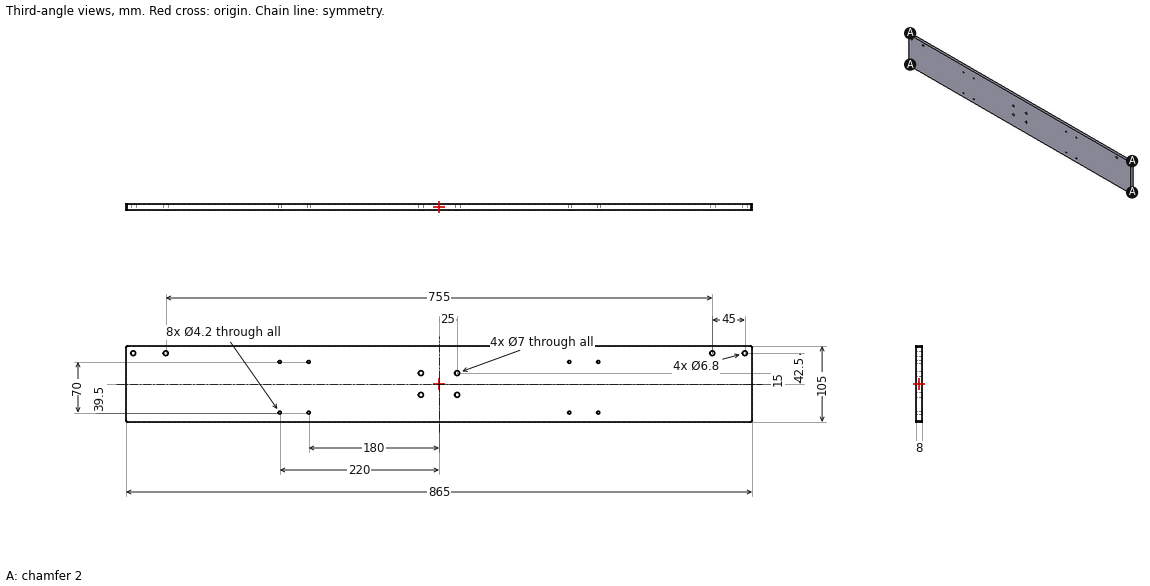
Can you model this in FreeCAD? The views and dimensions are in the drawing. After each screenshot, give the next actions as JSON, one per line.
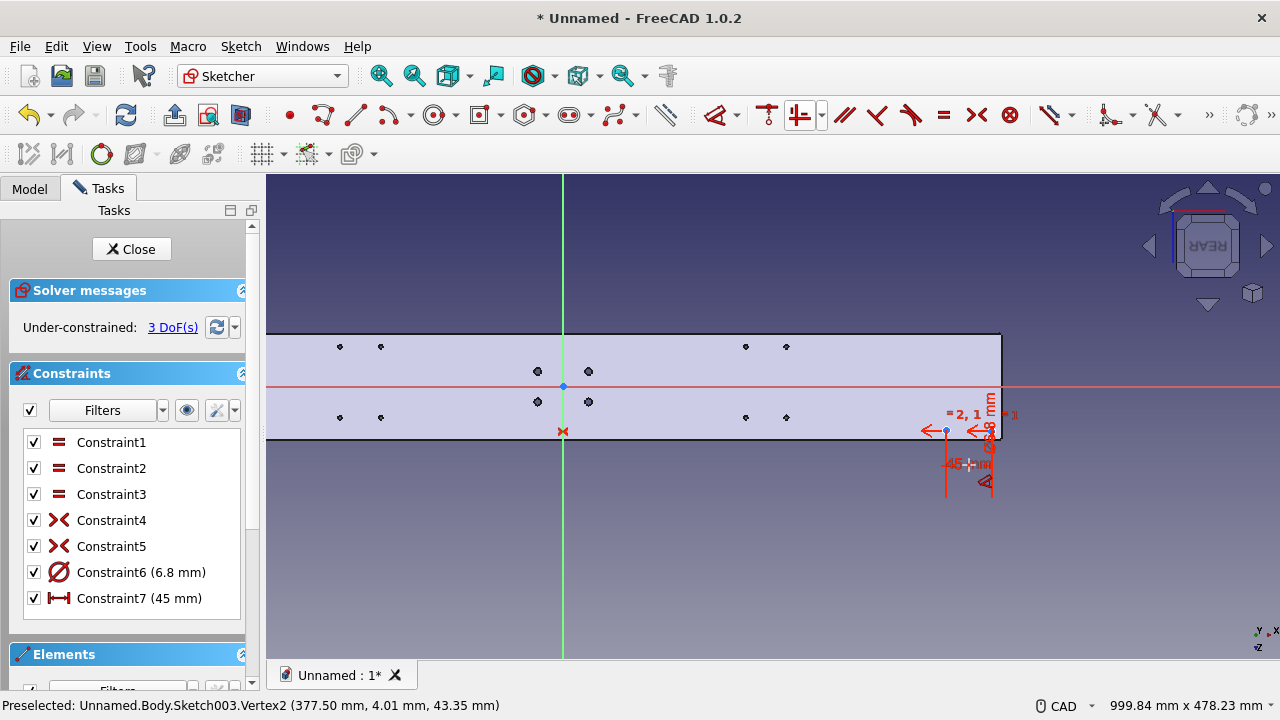
{"action": "left_click", "coordinate": [992, 431]}
{"action": "left_click", "coordinate": [529, 409]}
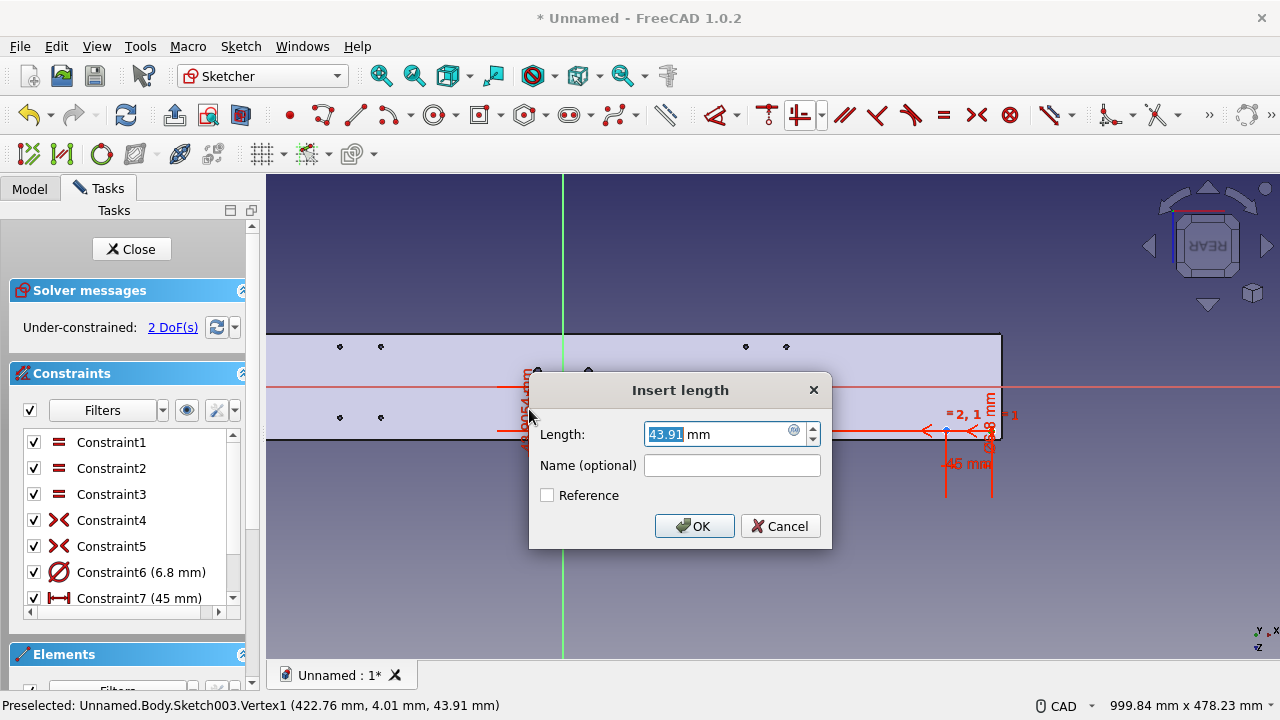
{"action": "type", "text": "42.5"}
{"action": "key", "text": "Return"}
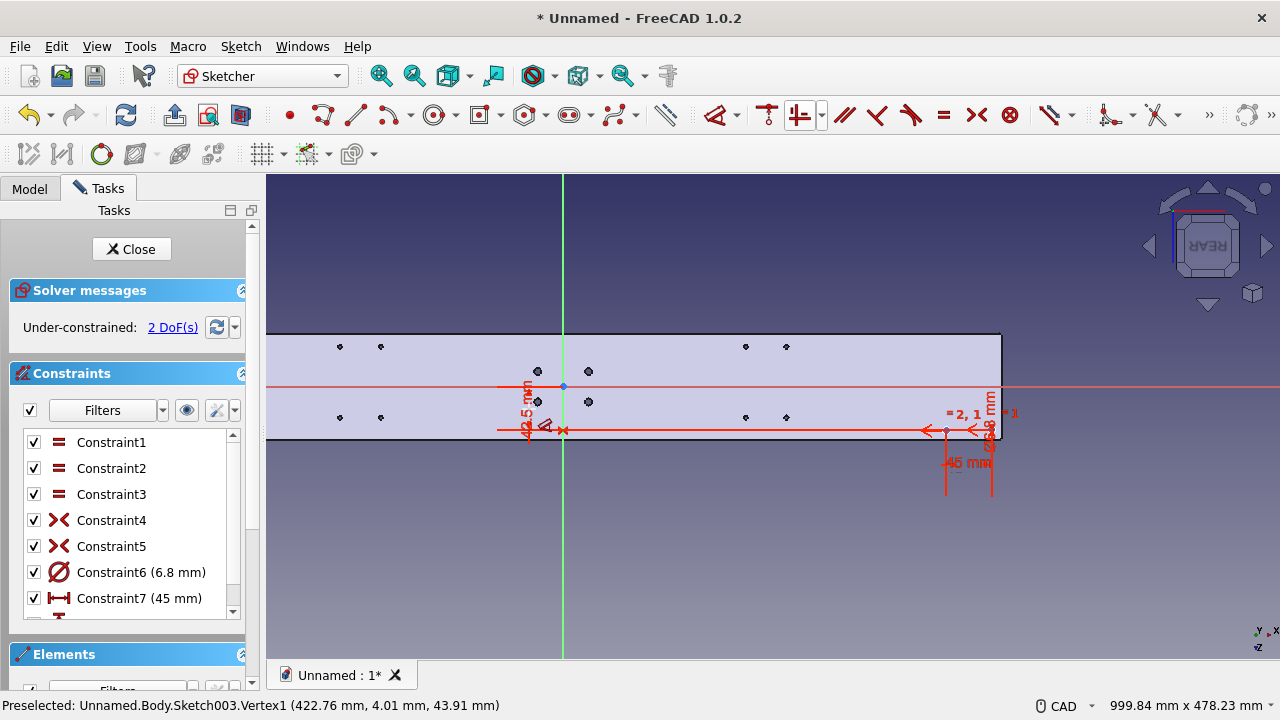
{"action": "left_click", "coordinate": [946, 431]}
{"action": "left_click", "coordinate": [457, 409]}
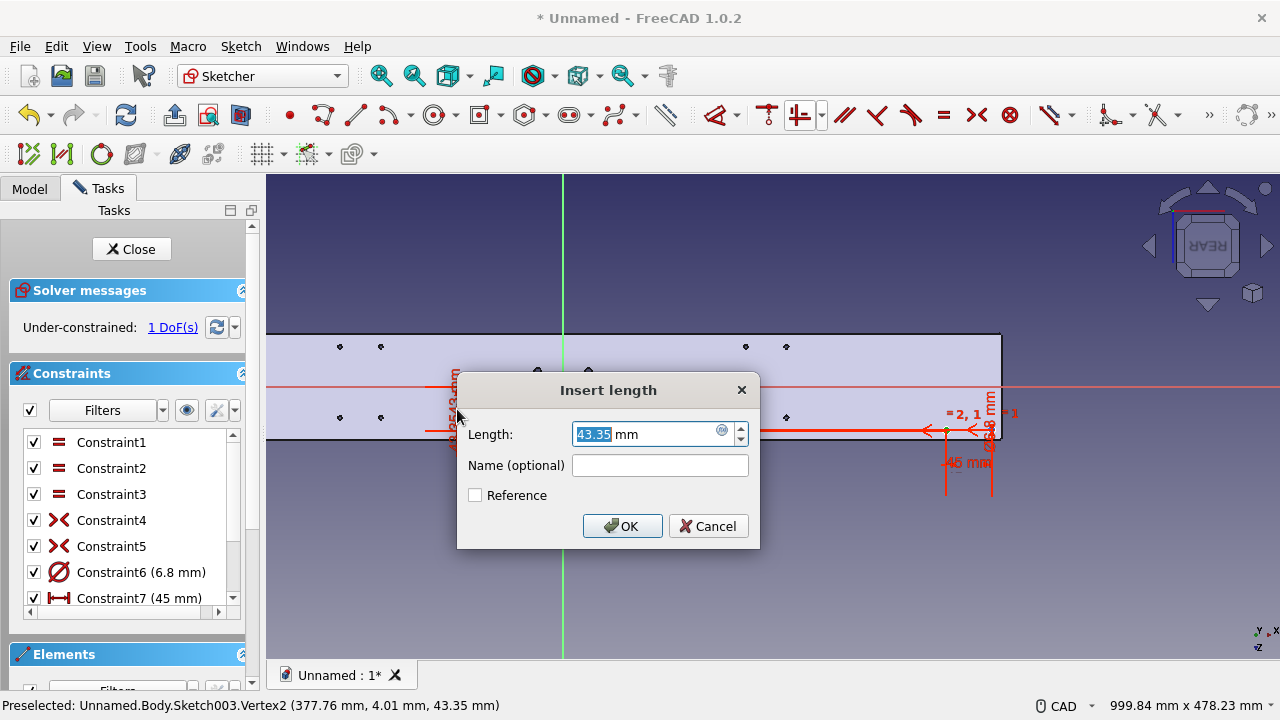
{"action": "type", "text": "42.5"}
{"action": "key", "text": "Return"}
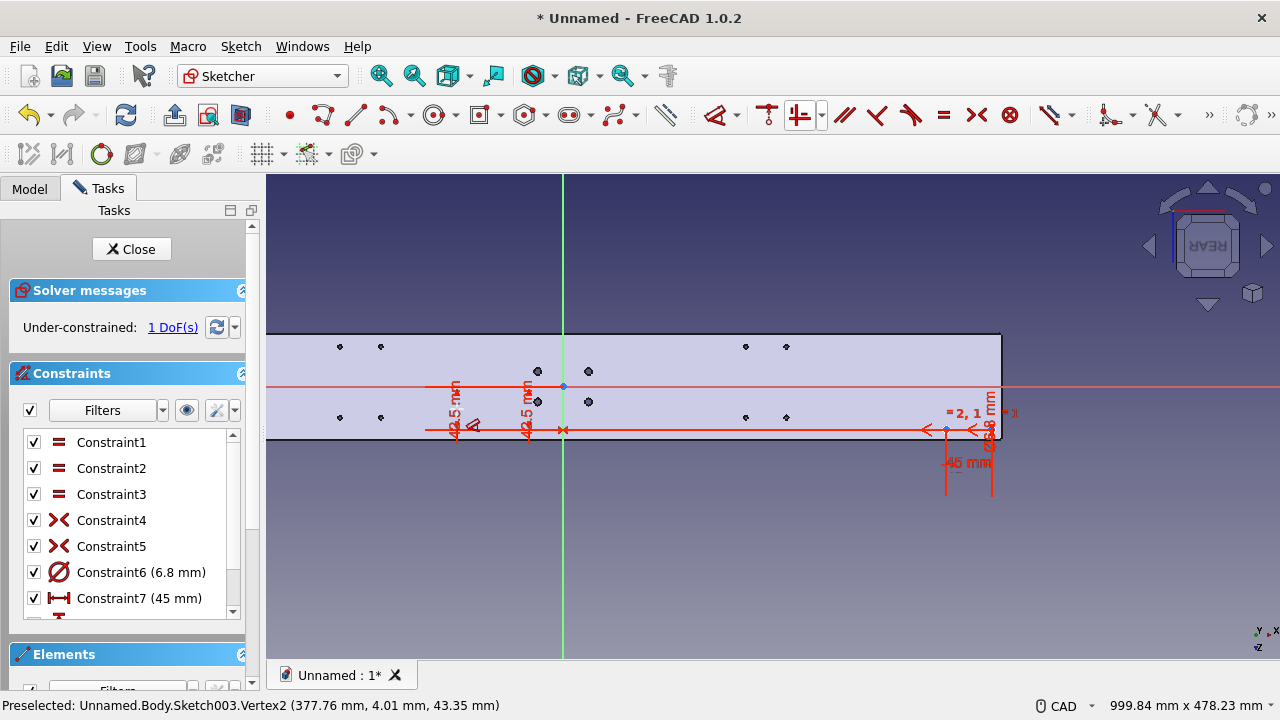
{"action": "left_click", "coordinate": [946, 430]}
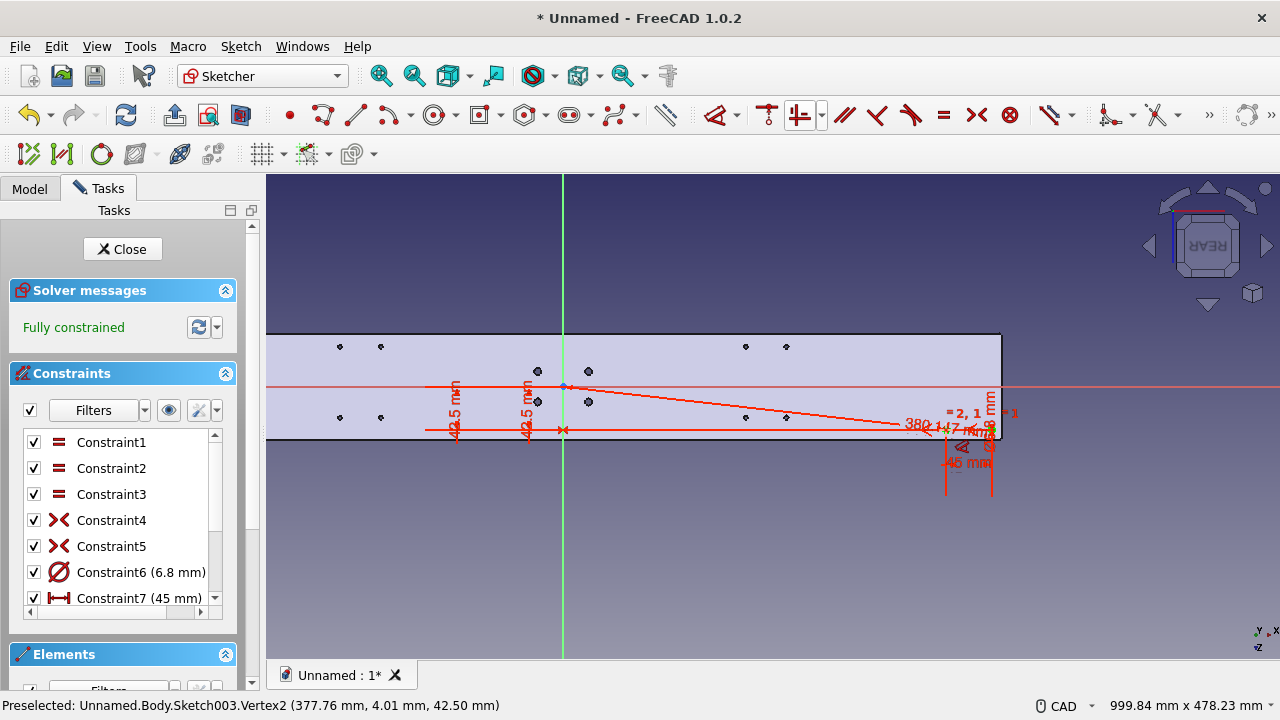
{"action": "scroll", "coordinate": [992, 430], "scroll_direction": "down", "scroll_amount": 2}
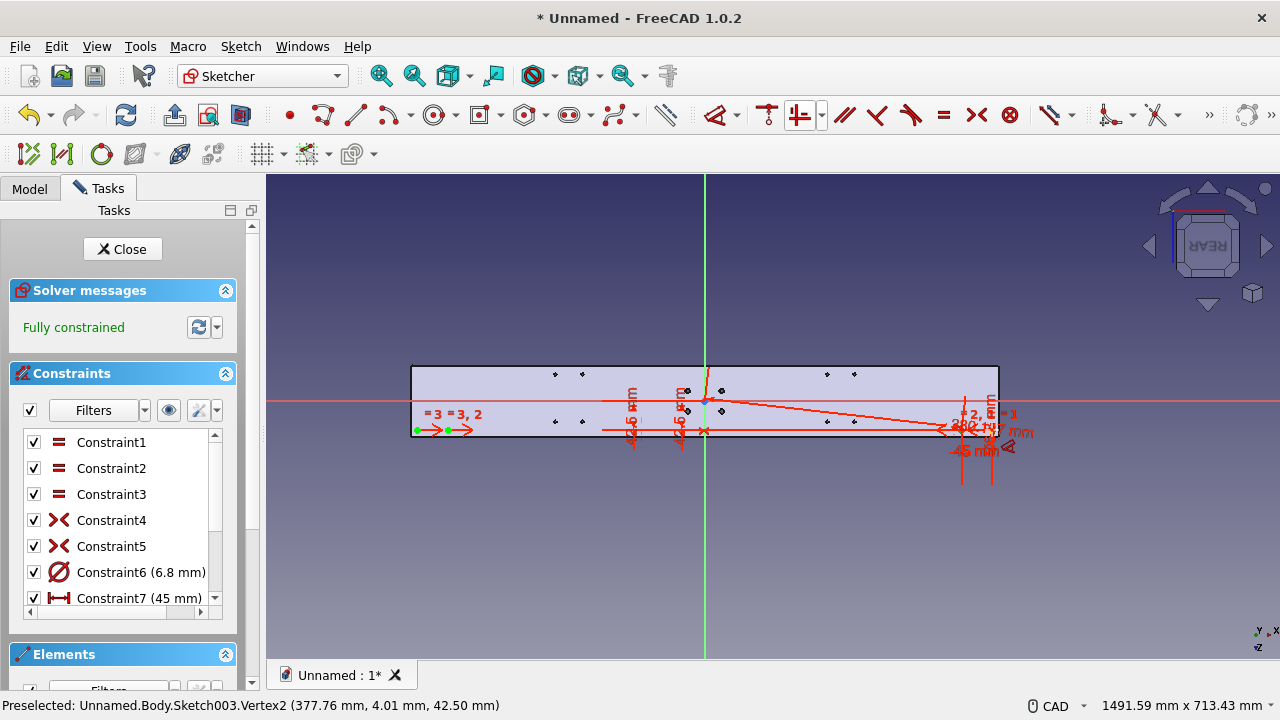
{"action": "left_click", "coordinate": [448, 430]}
{"action": "left_click", "coordinate": [587, 464]}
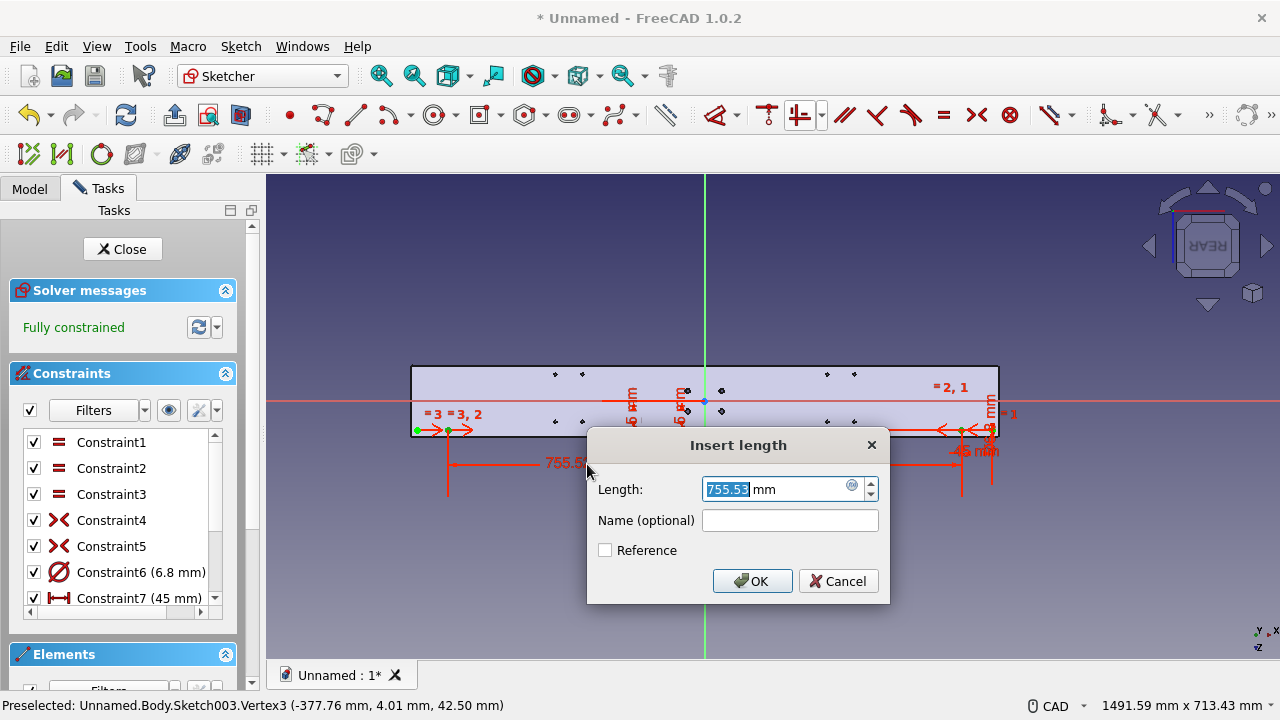
{"action": "type", "text": "755"}
{"action": "key", "text": "Return"}
{"action": "key", "text": "Escape"}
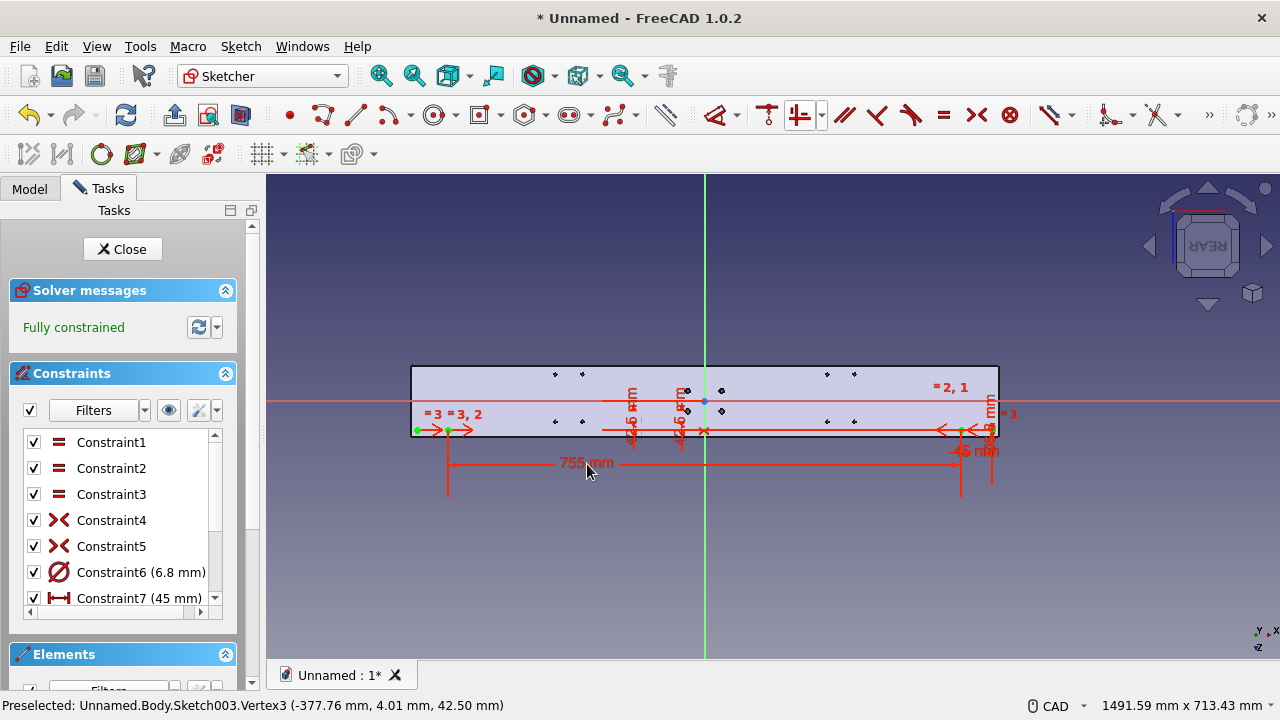
{"action": "left_click", "coordinate": [123, 249]}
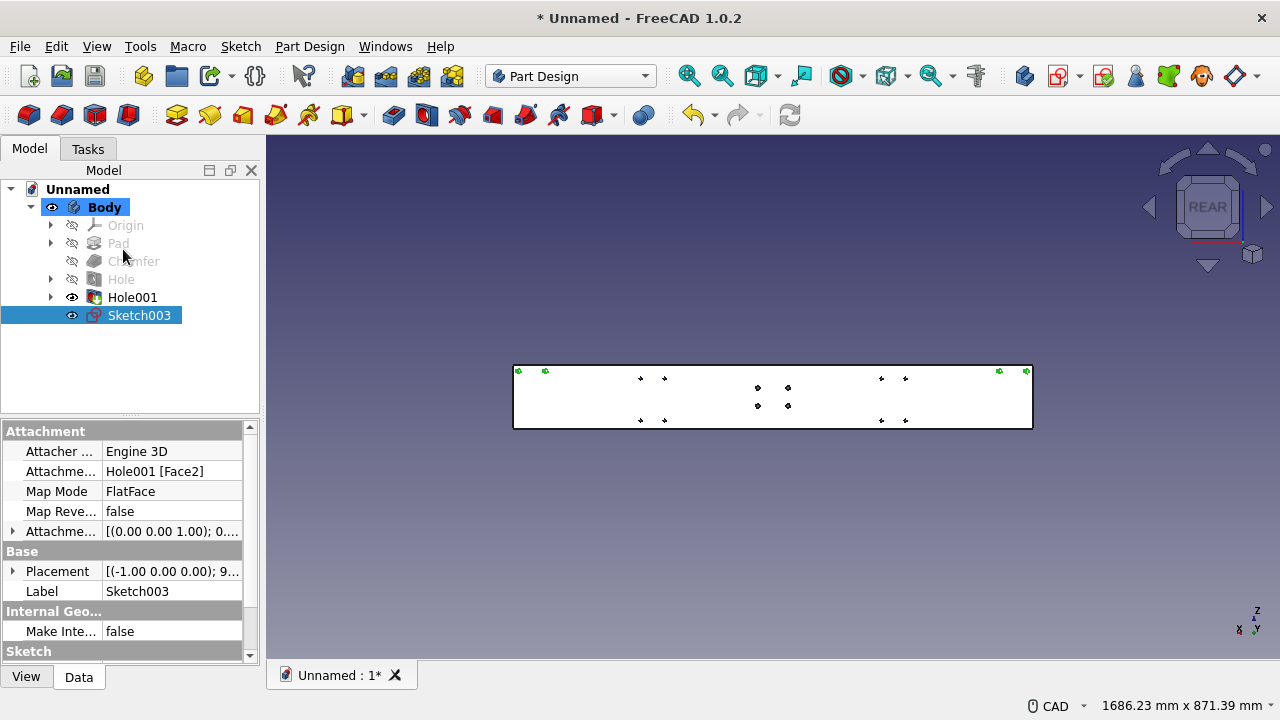
{"action": "left_click", "coordinate": [394, 116]}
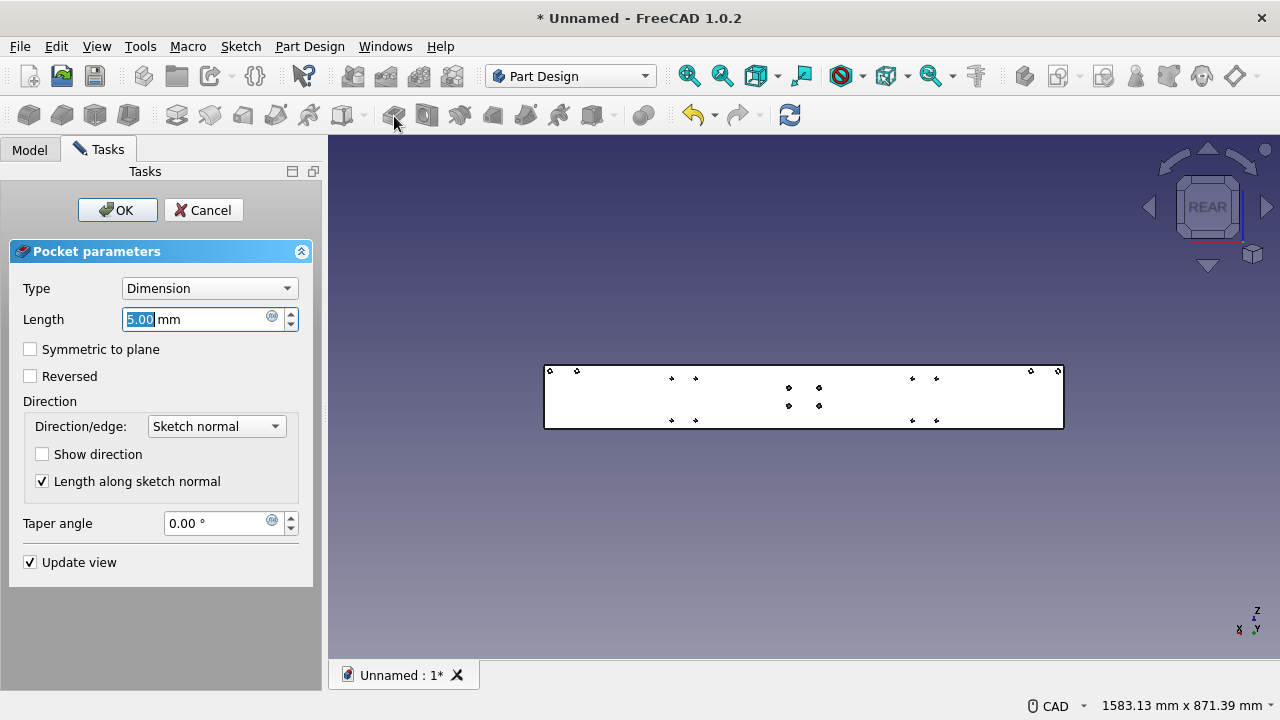
{"action": "left_click", "coordinate": [210, 288]}